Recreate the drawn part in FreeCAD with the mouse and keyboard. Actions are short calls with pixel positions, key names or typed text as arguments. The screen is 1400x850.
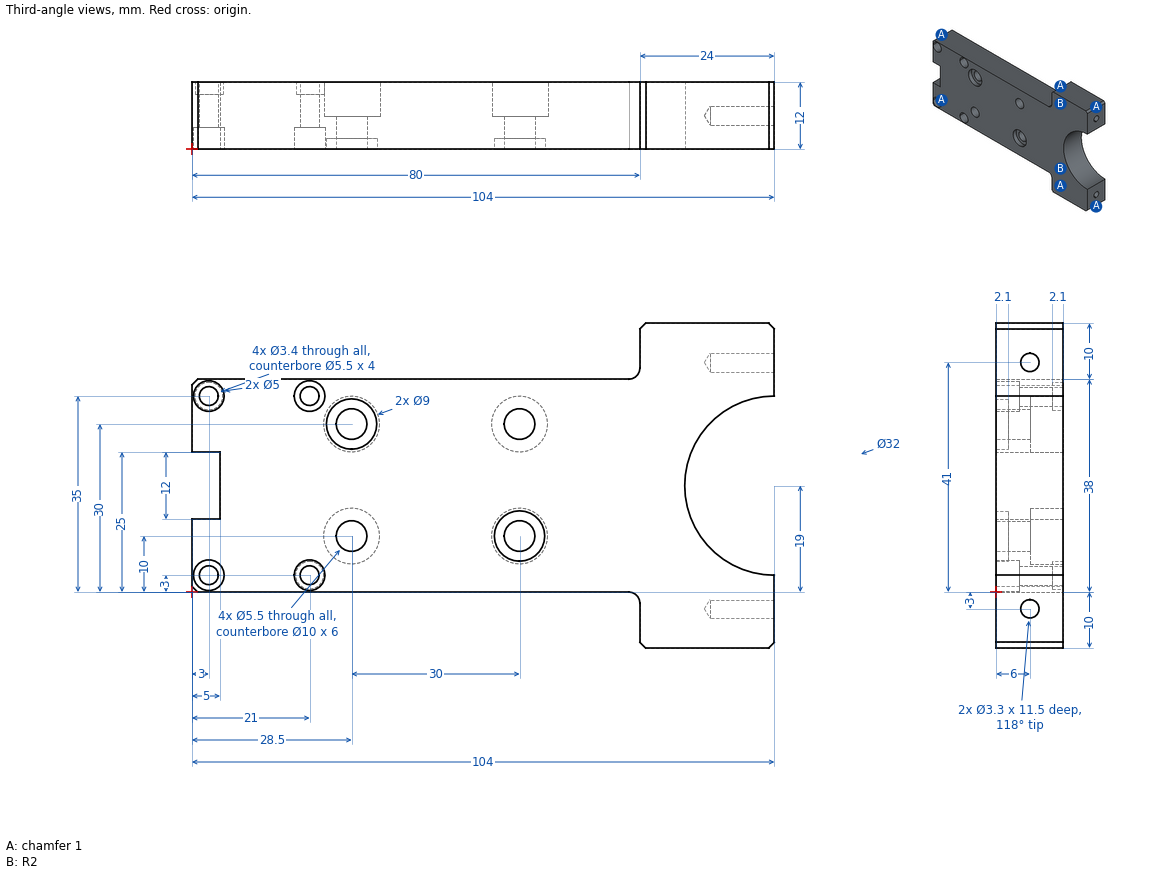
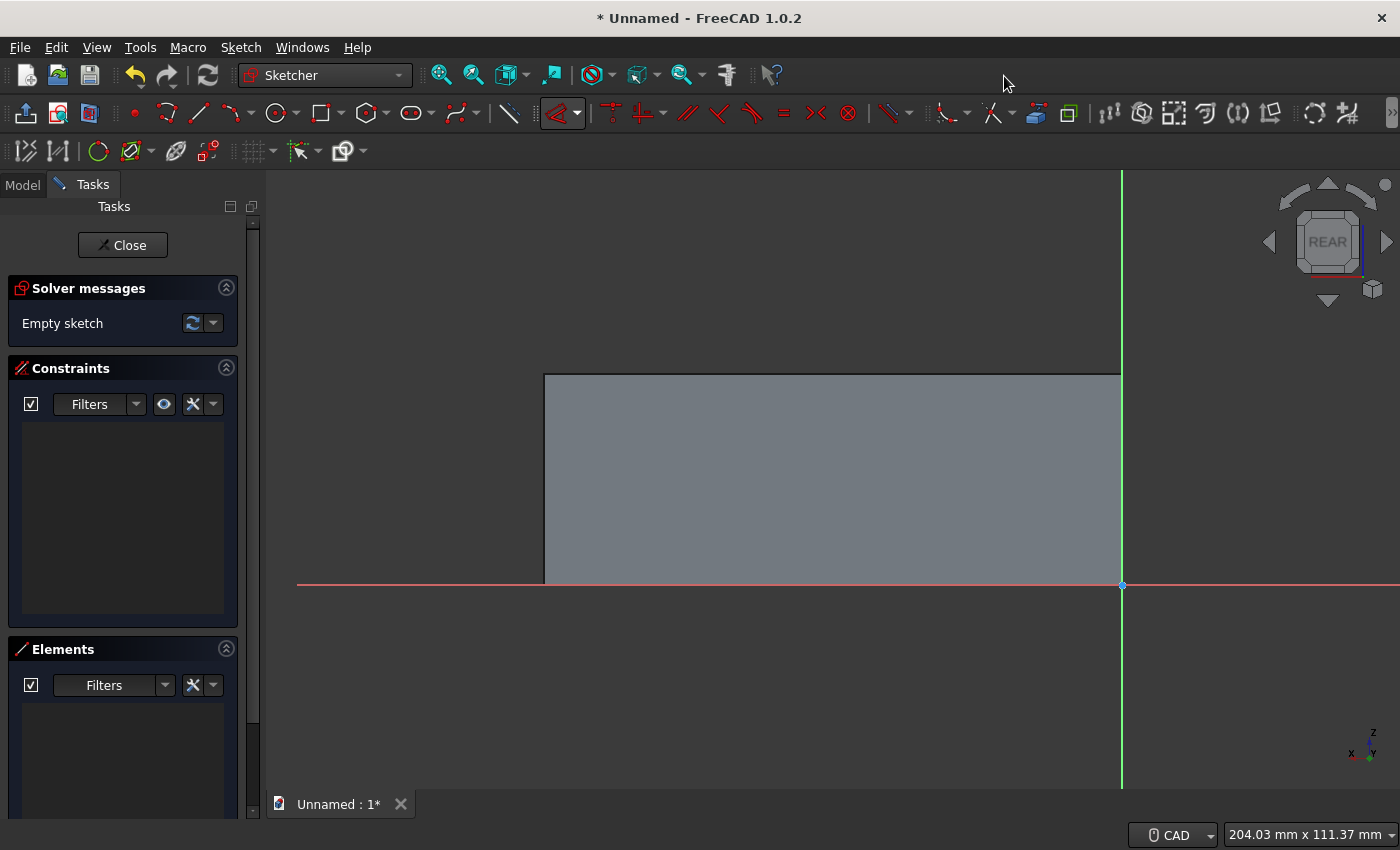
scroll(1235, 537, up, 5)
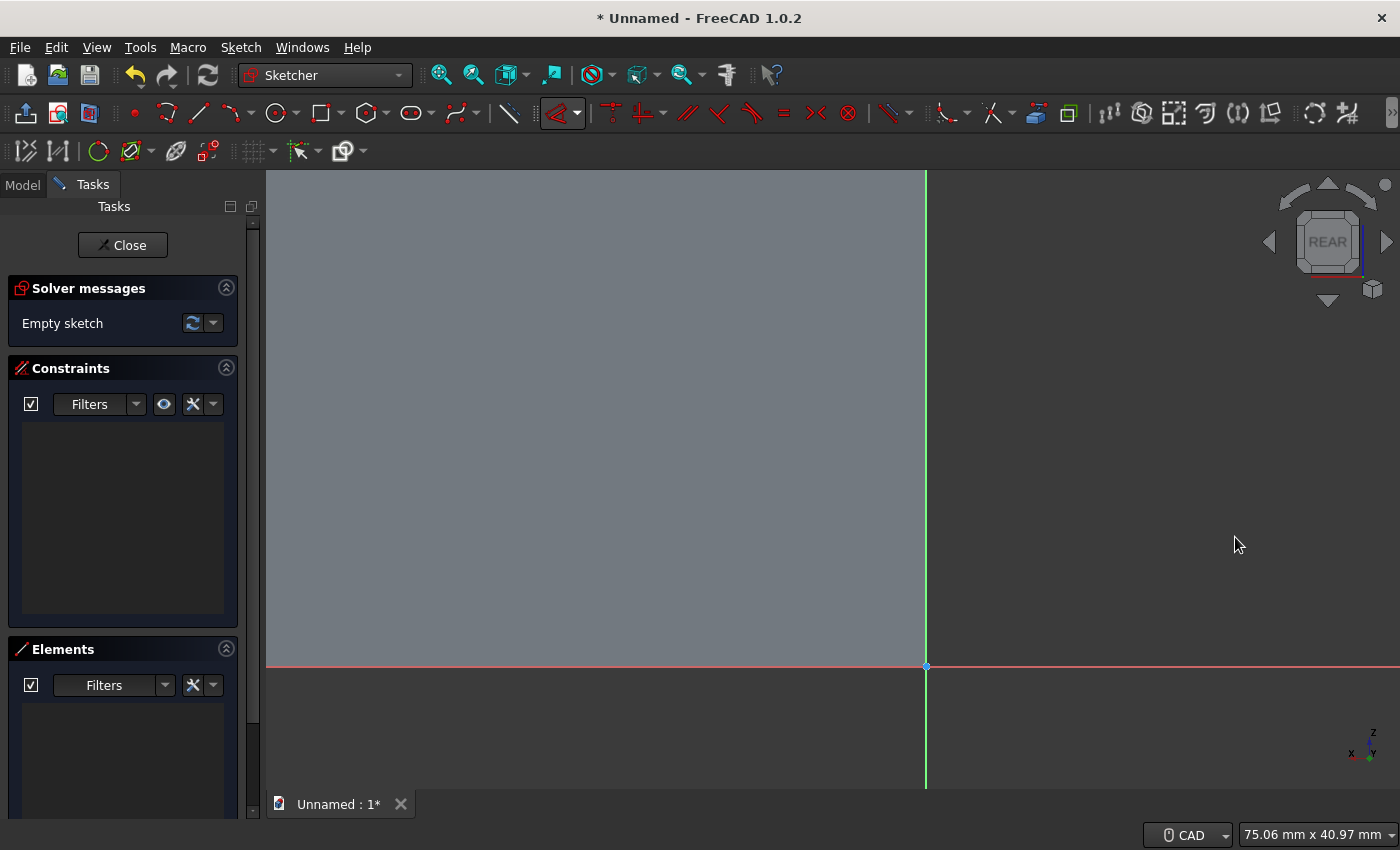
click(322, 114)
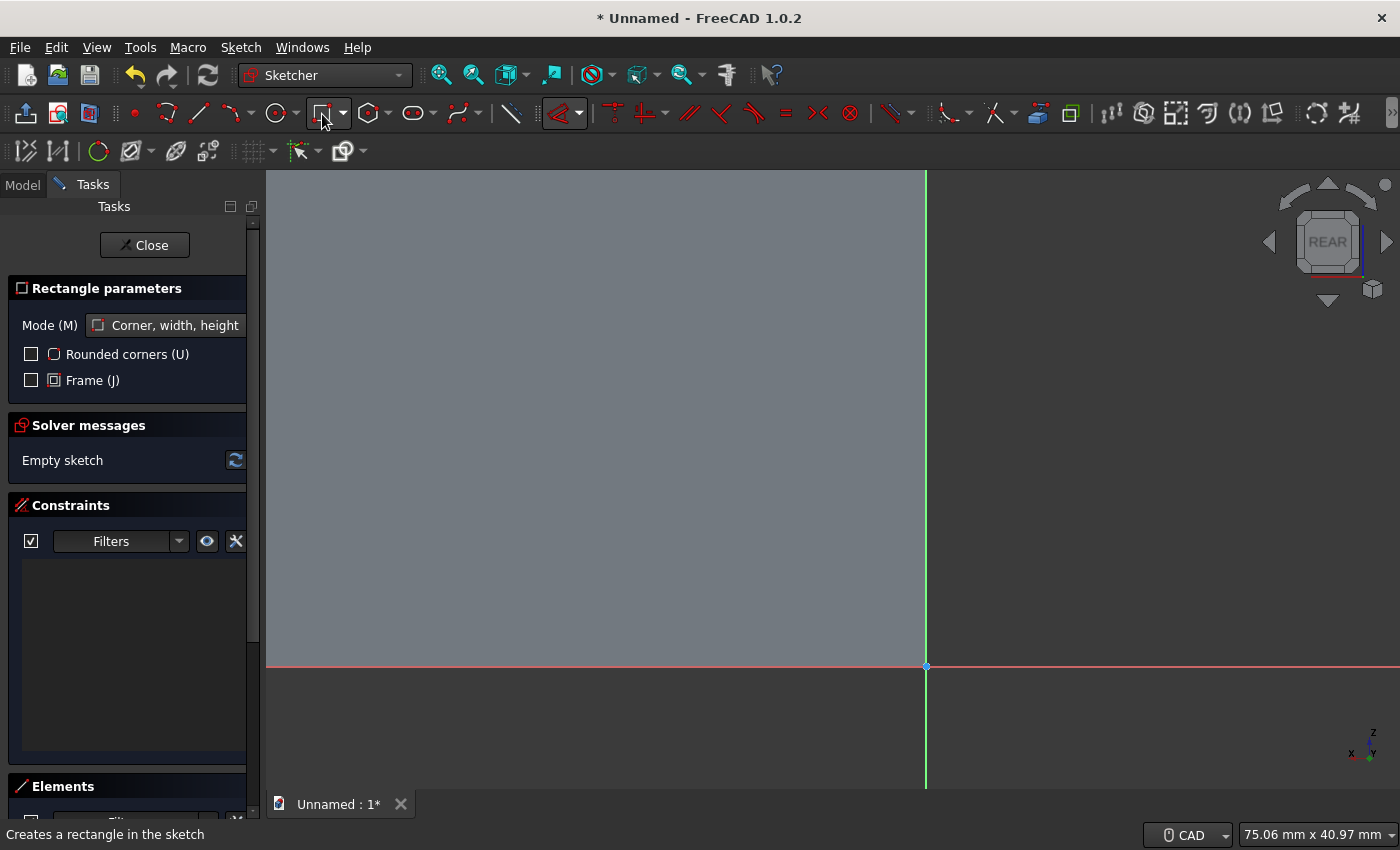
click(851, 289)
click(926, 470)
key(Escape)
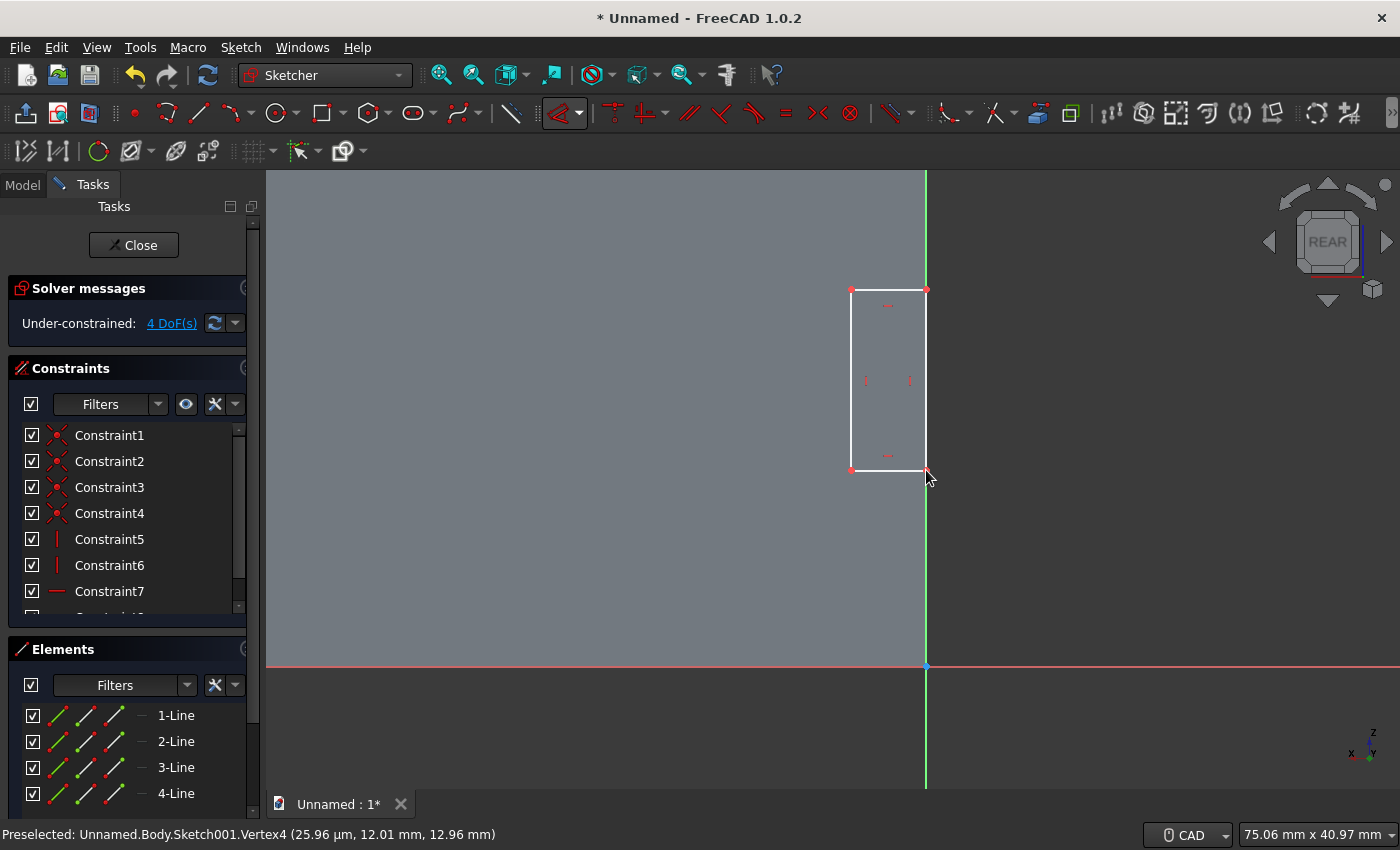
click(926, 471)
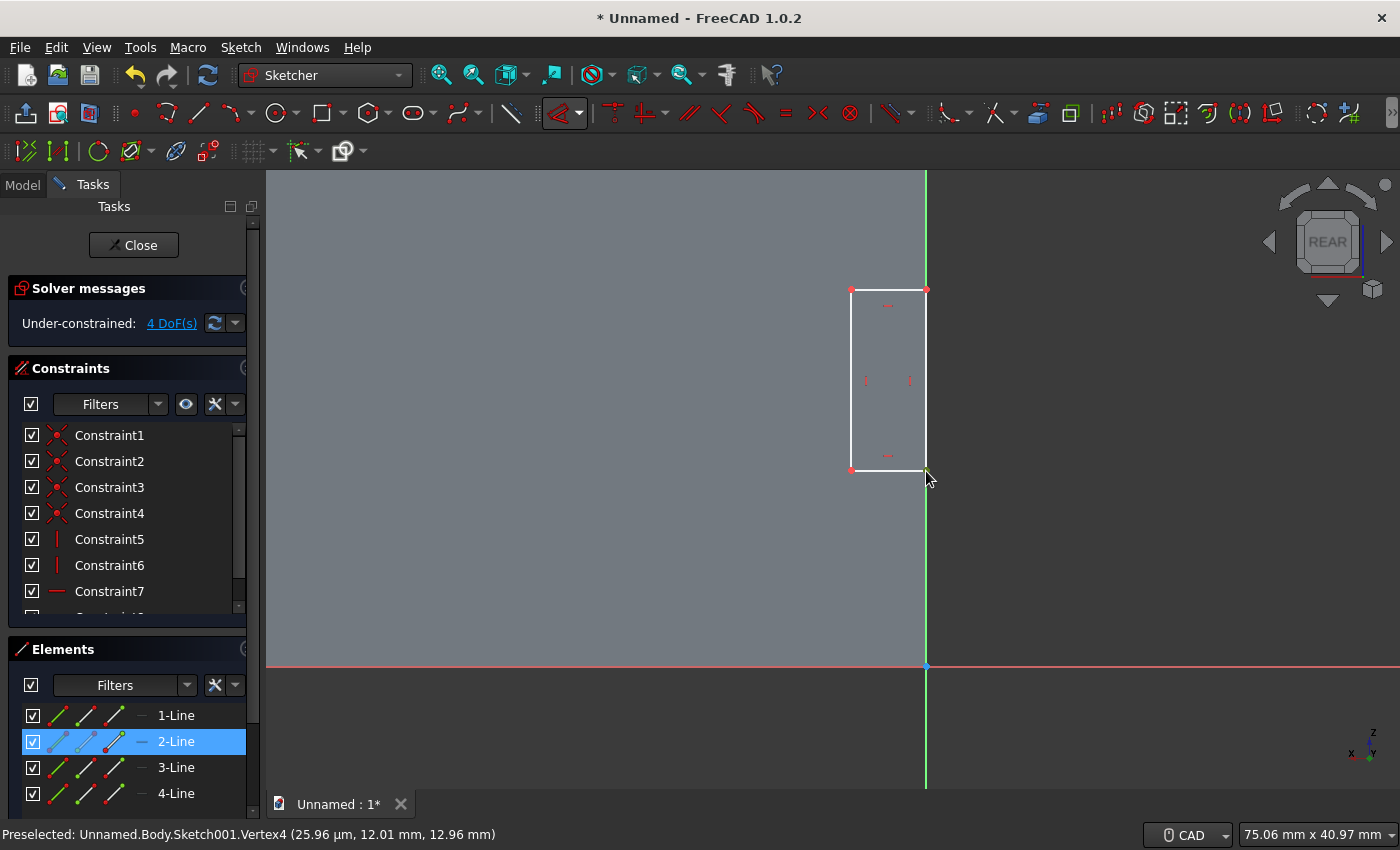
click(926, 721)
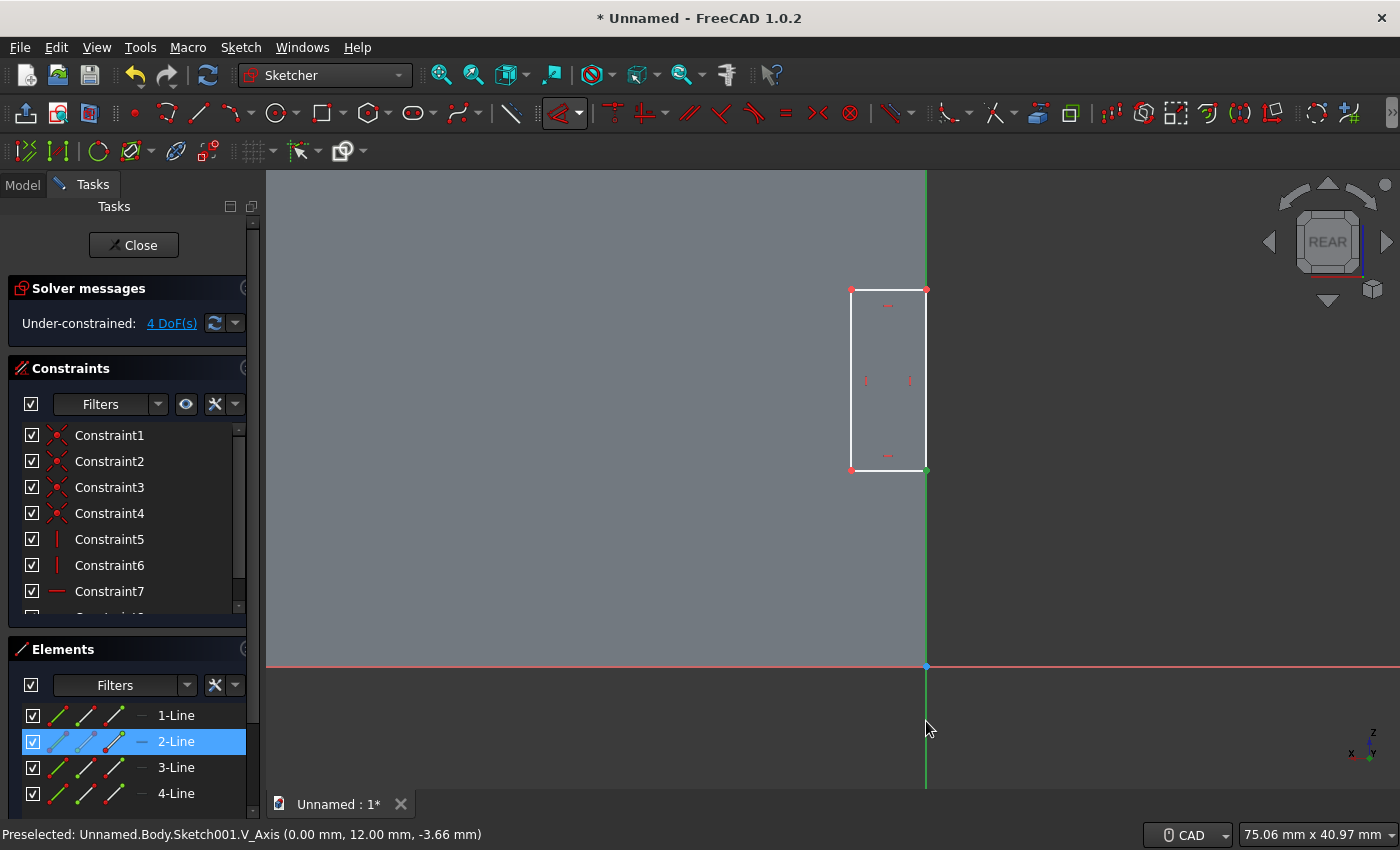
click(614, 114)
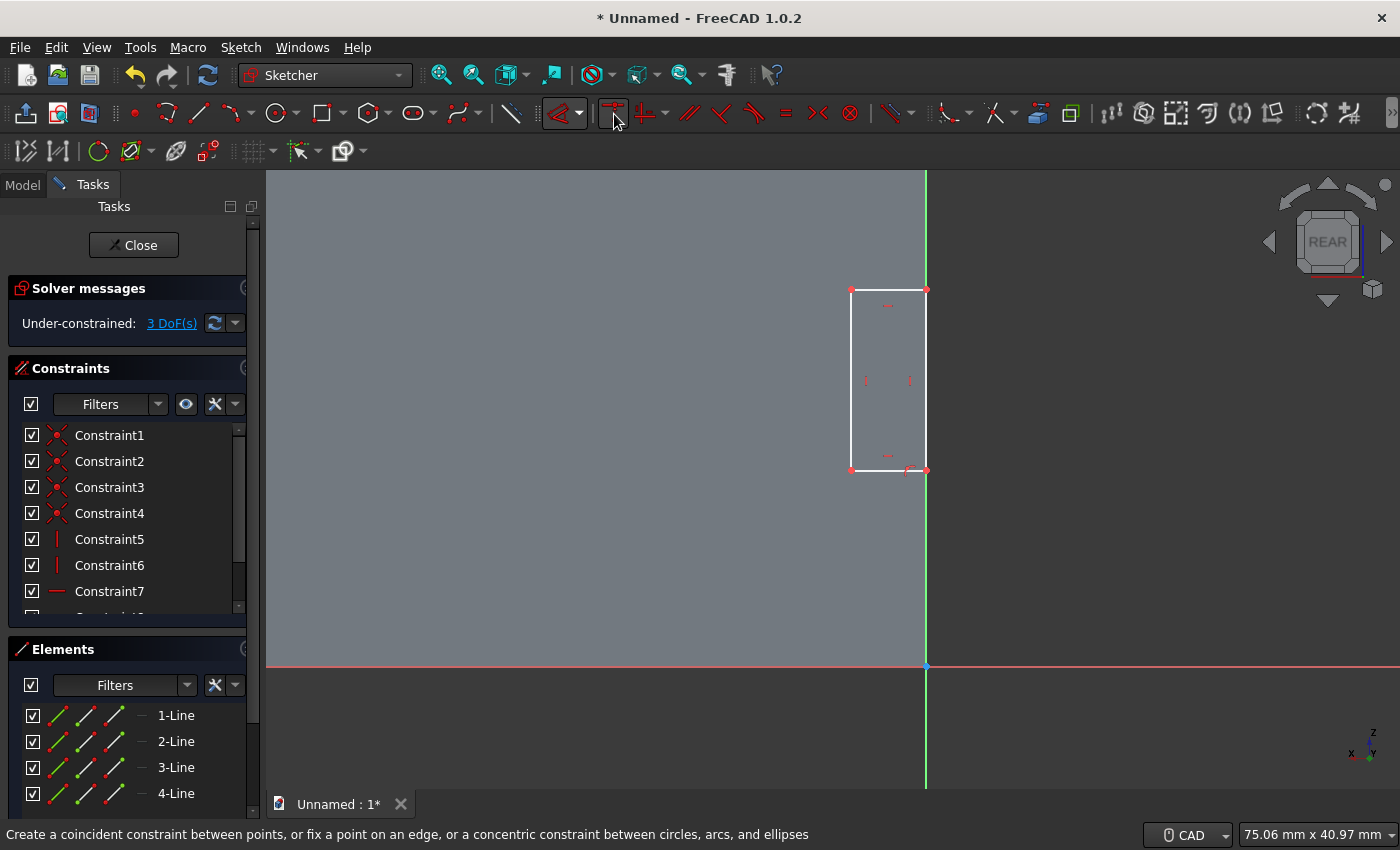
click(874, 471)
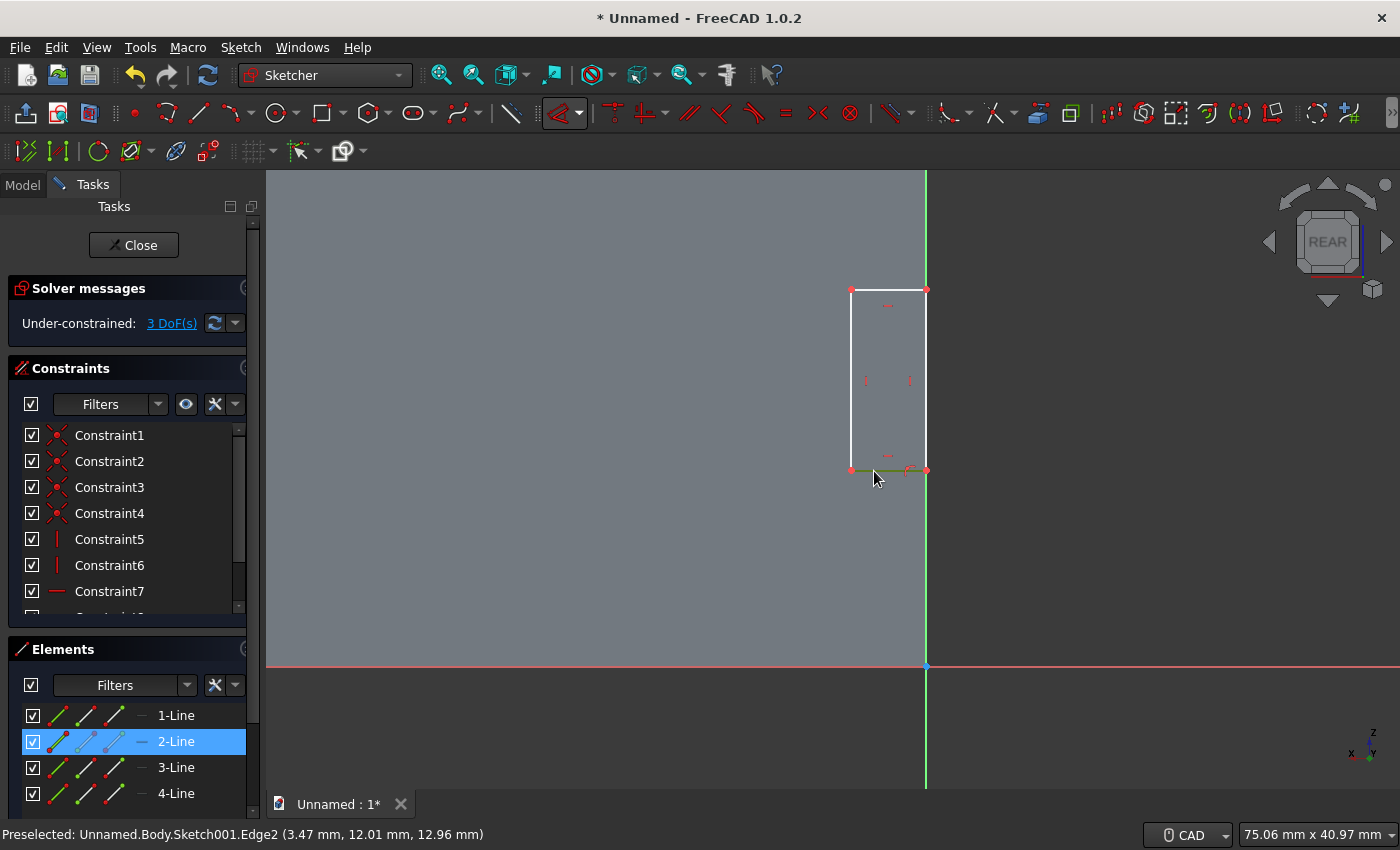
key(l)